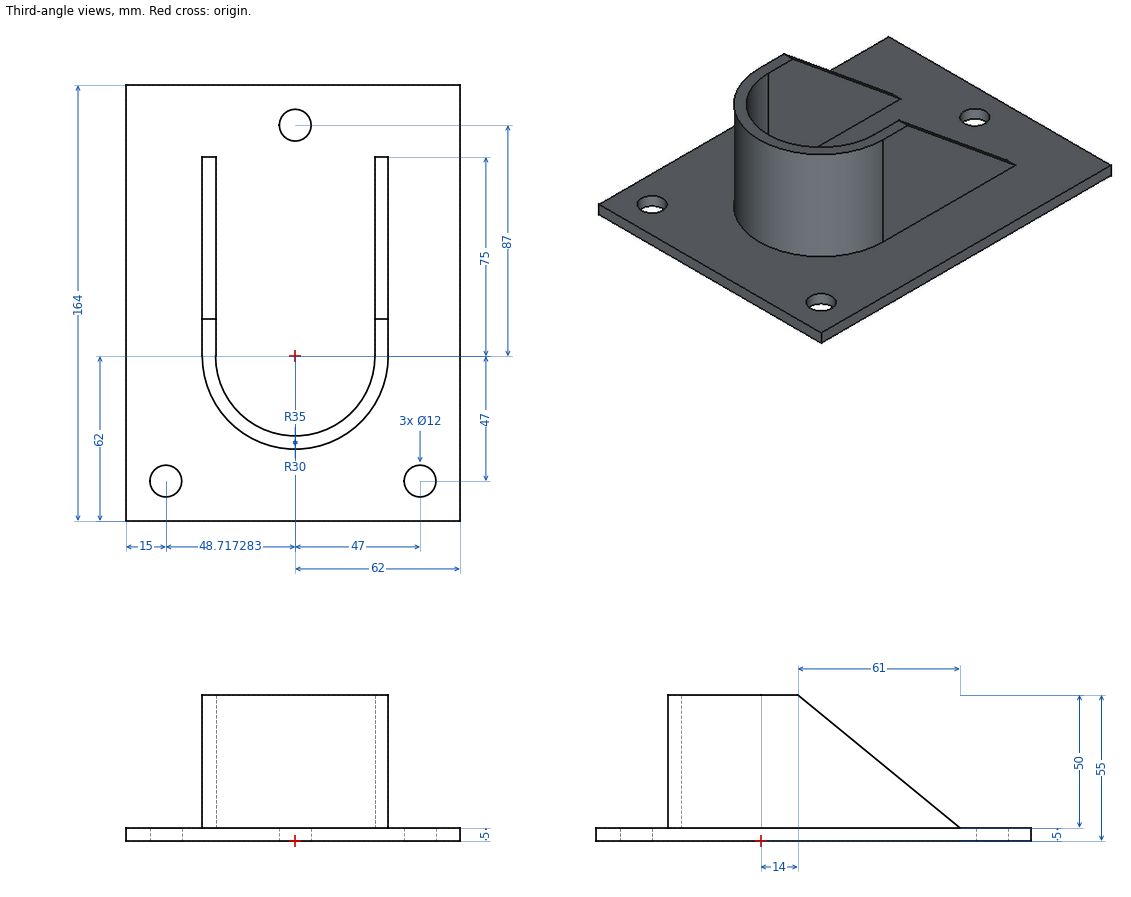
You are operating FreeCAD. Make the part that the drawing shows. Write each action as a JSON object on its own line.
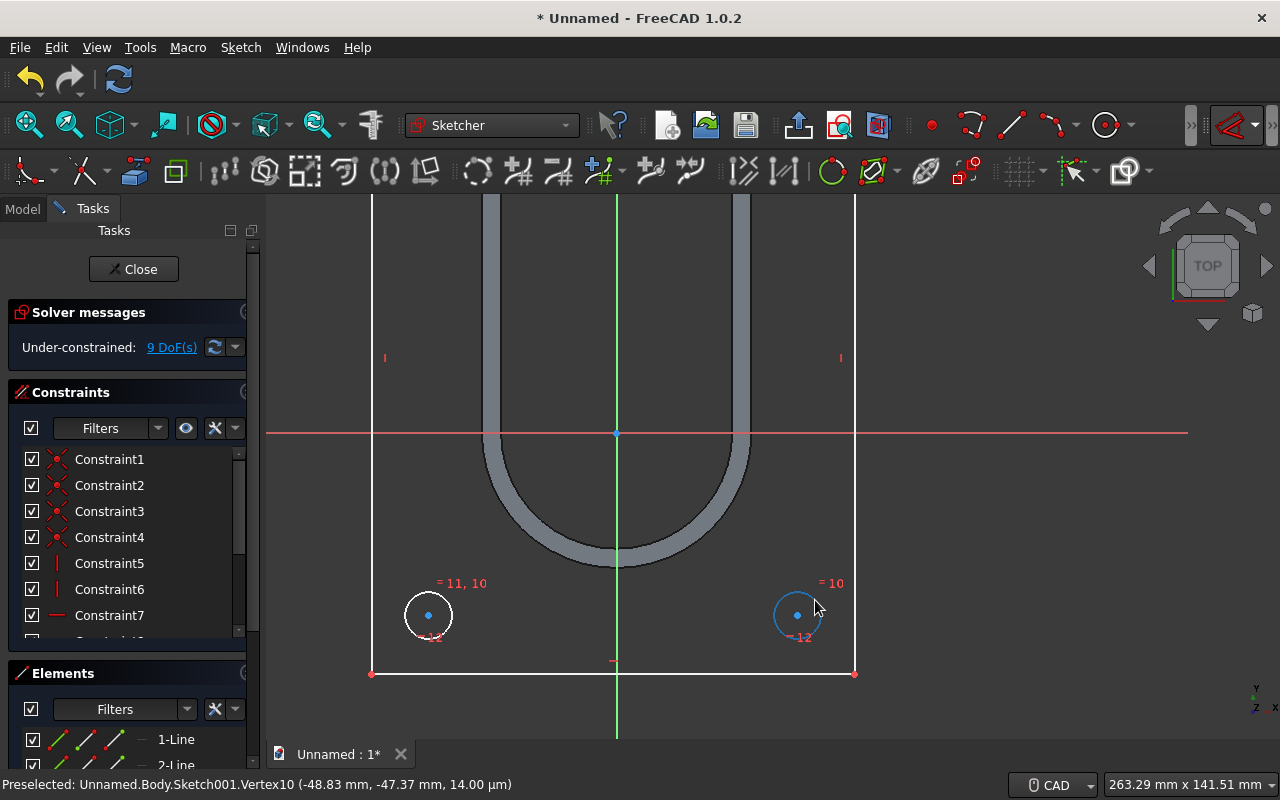
{"action": "left_click", "coordinate": [814, 599]}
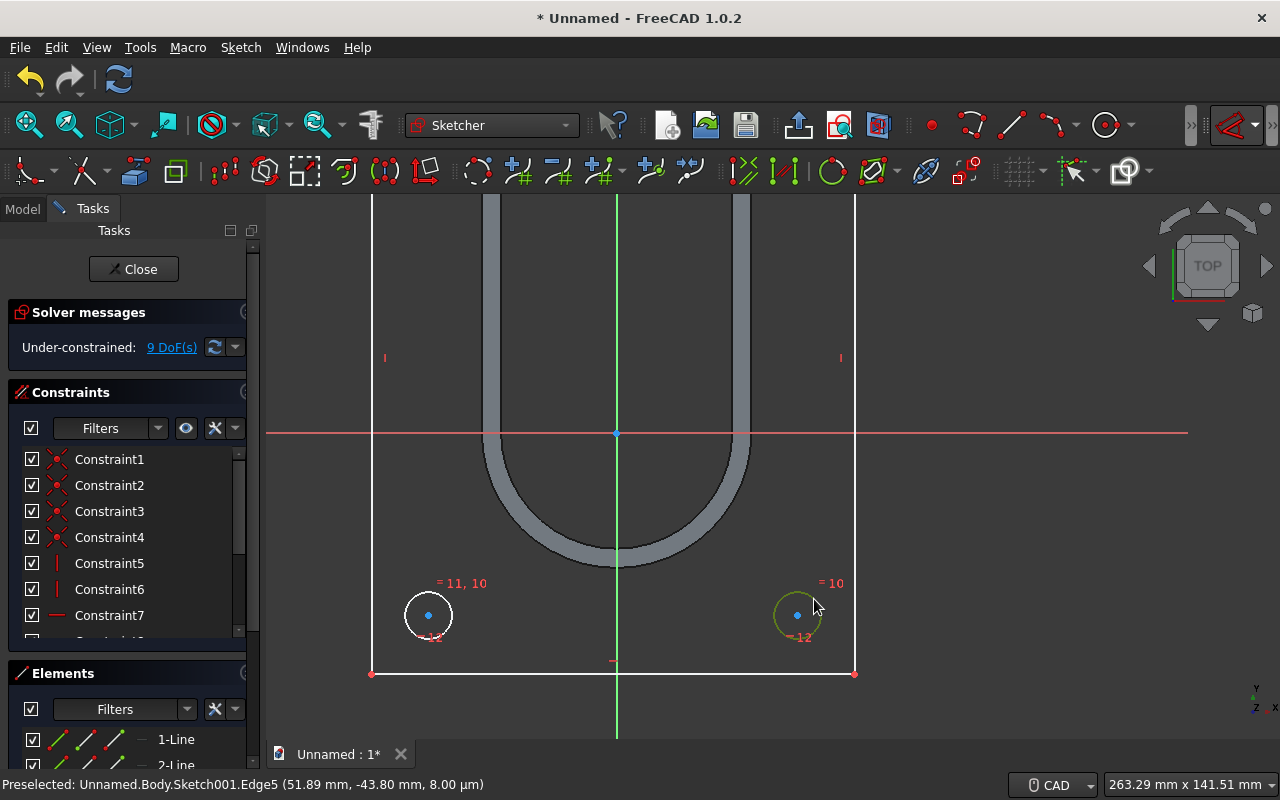
{"action": "left_click", "coordinate": [1258, 126]}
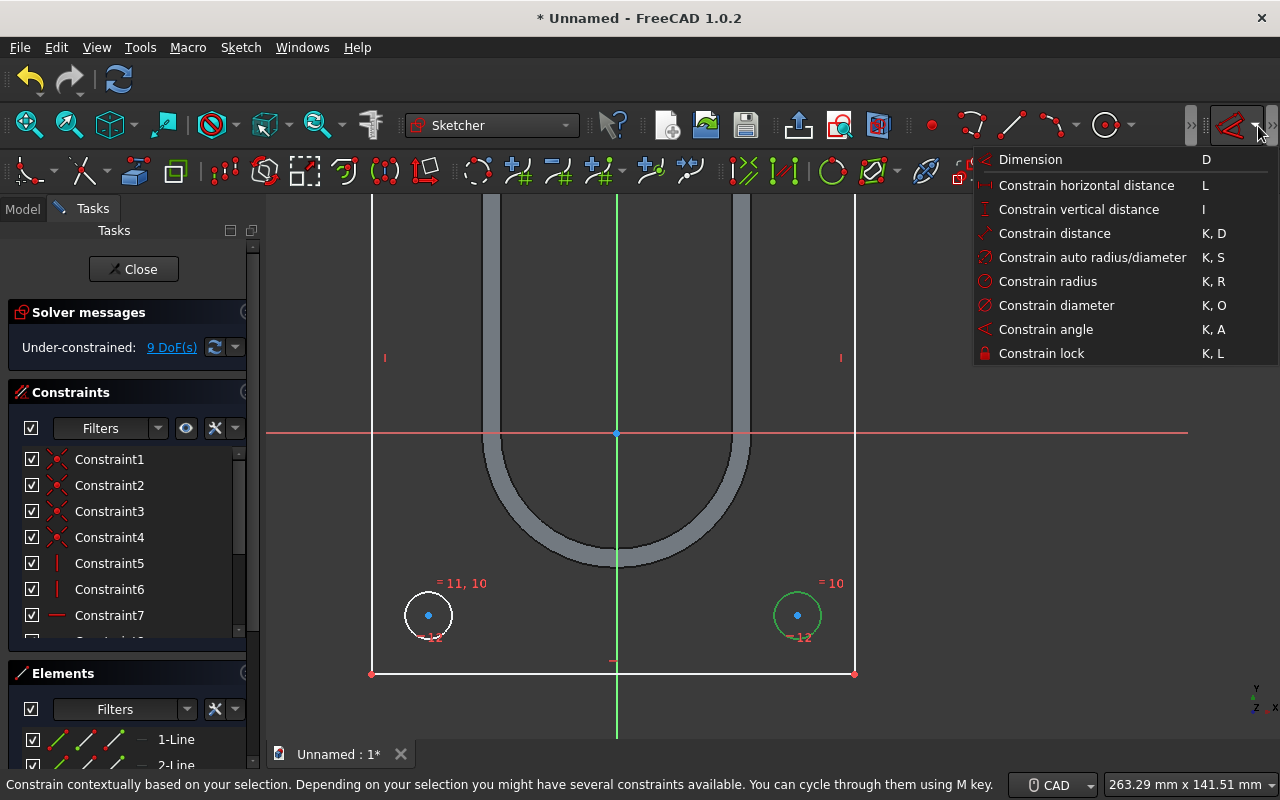
{"action": "left_click", "coordinate": [1126, 305]}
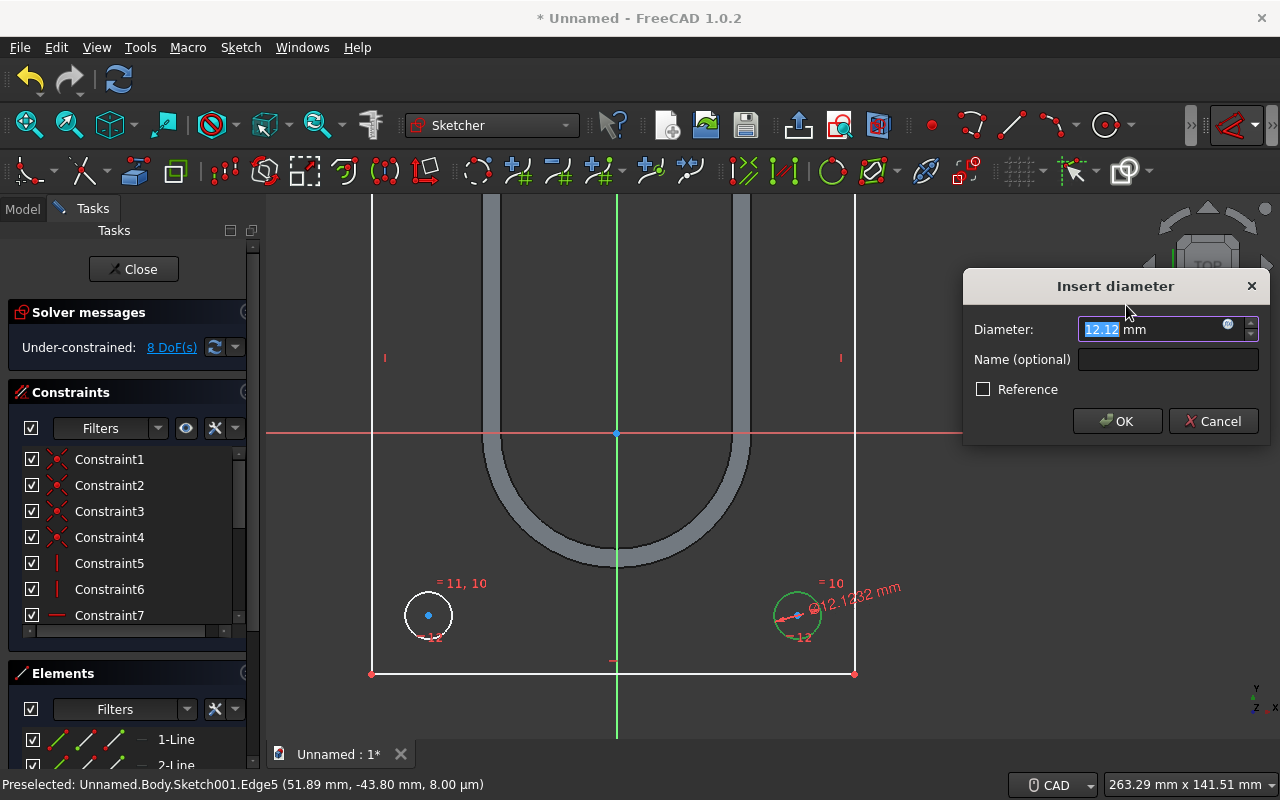
{"action": "type", "text": "12"}
{"action": "key", "text": "Return"}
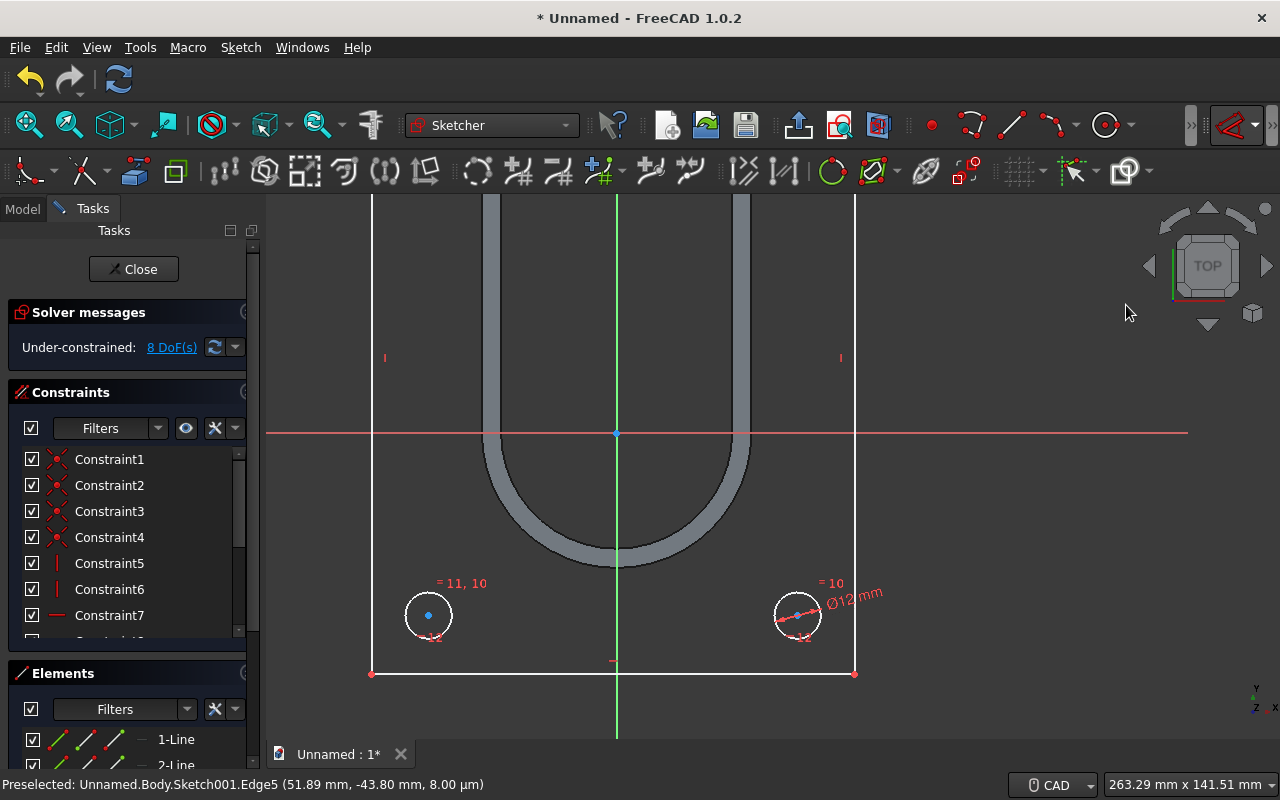
{"action": "left_click", "coordinate": [798, 616]}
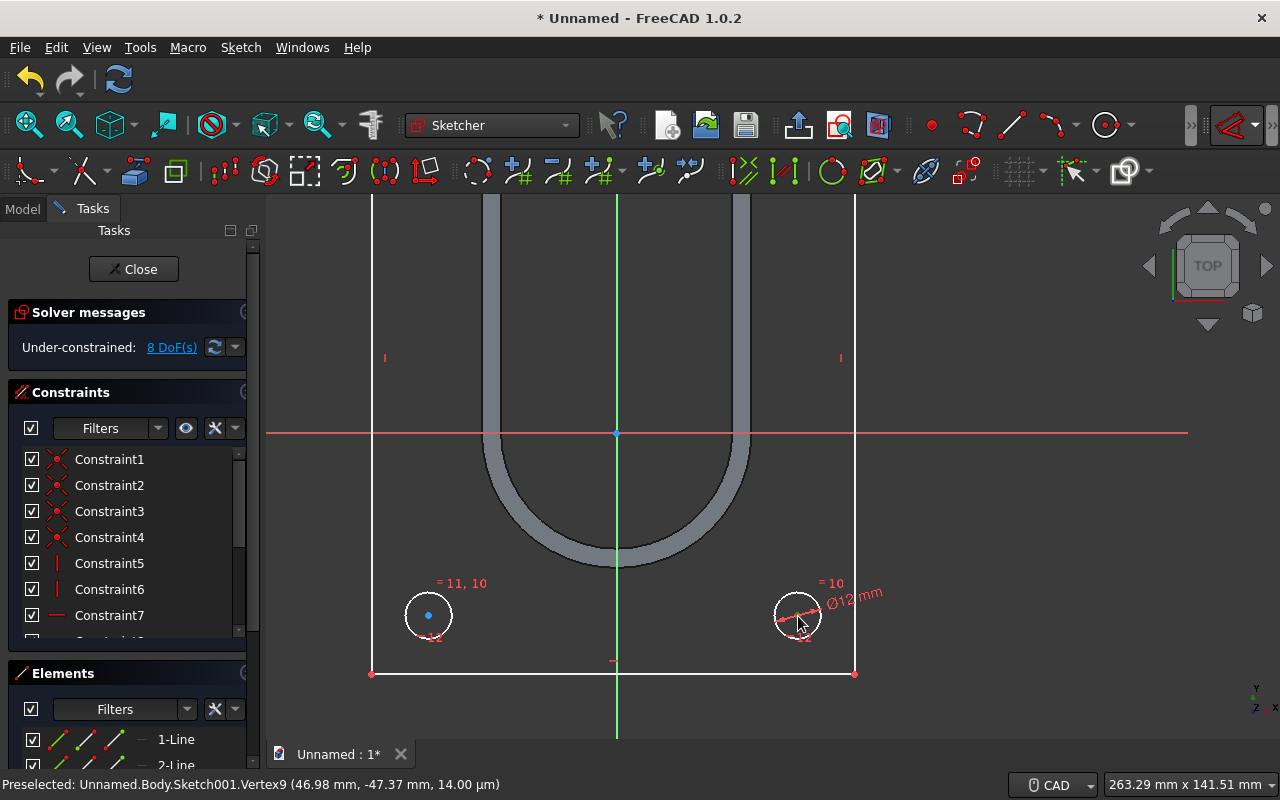
{"action": "key", "text": "l"}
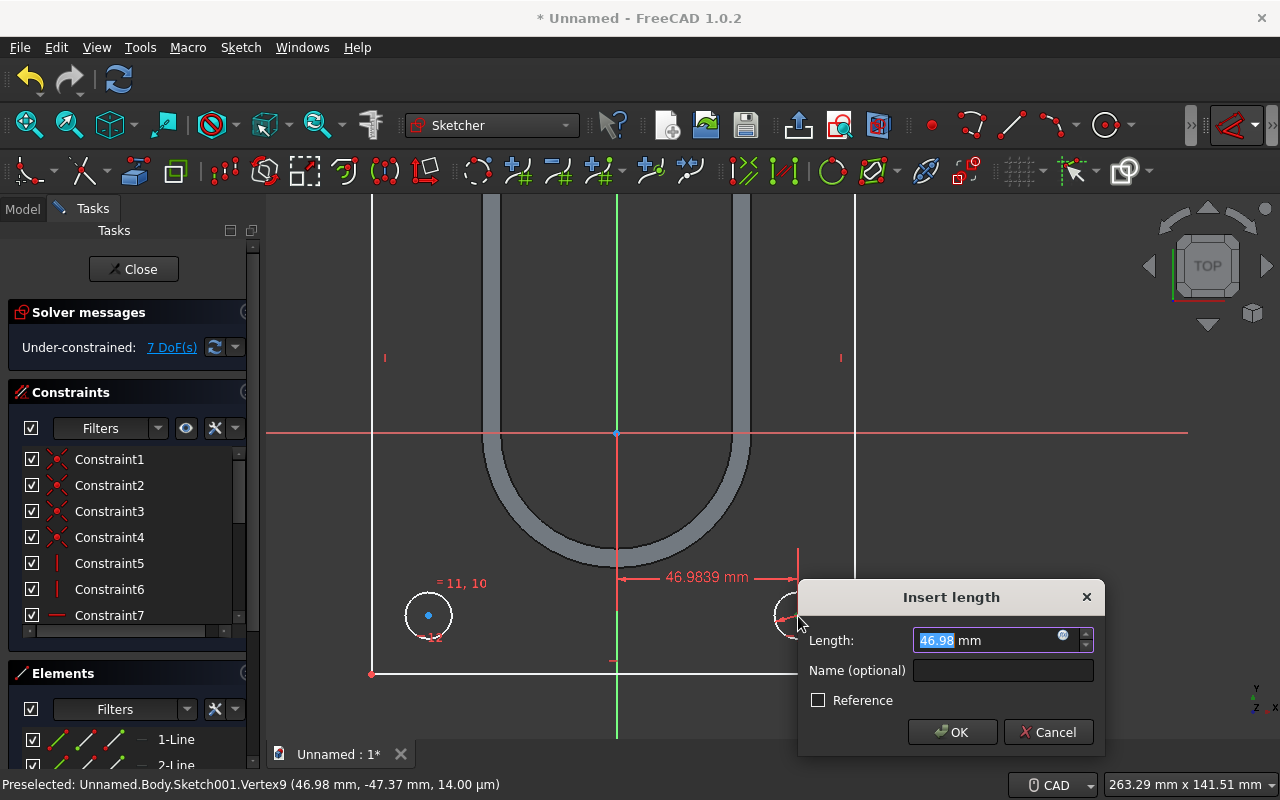
{"action": "type", "text": "47"}
{"action": "key", "text": "Return"}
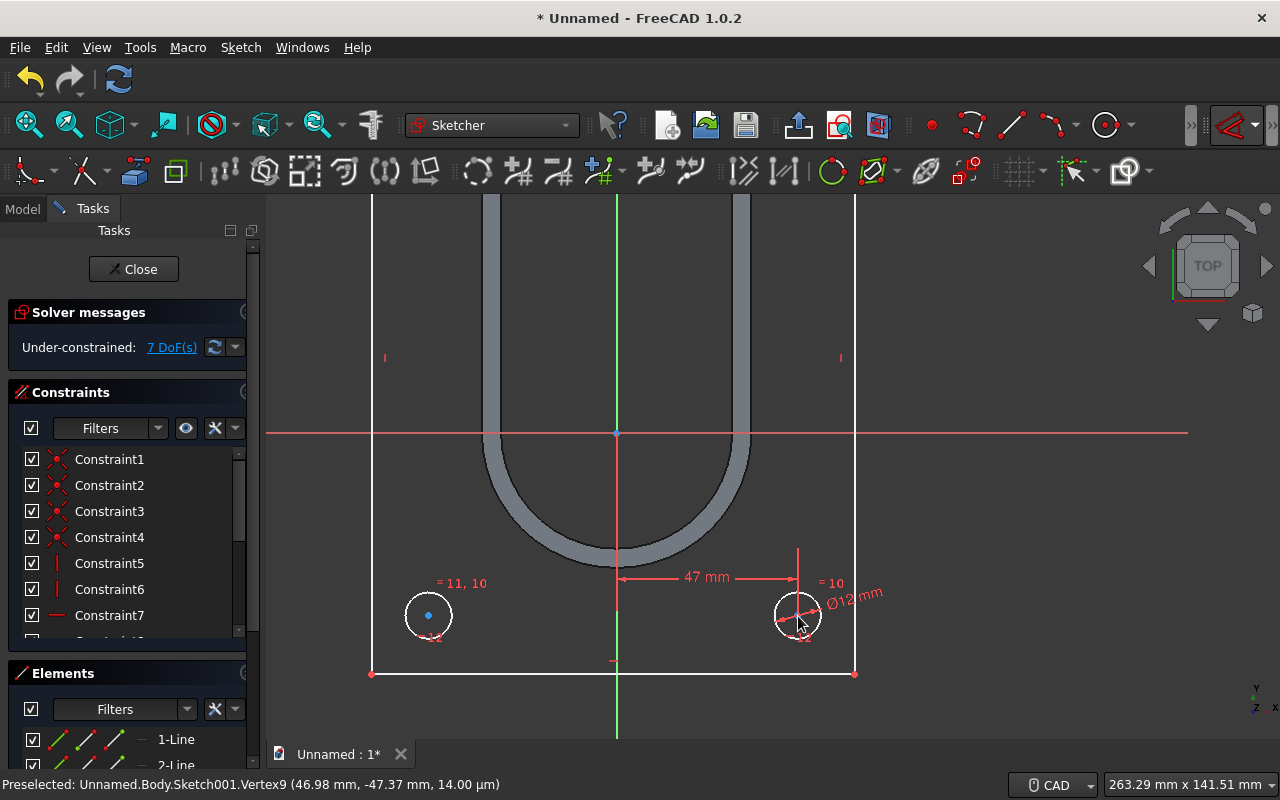
{"action": "left_click", "coordinate": [798, 616]}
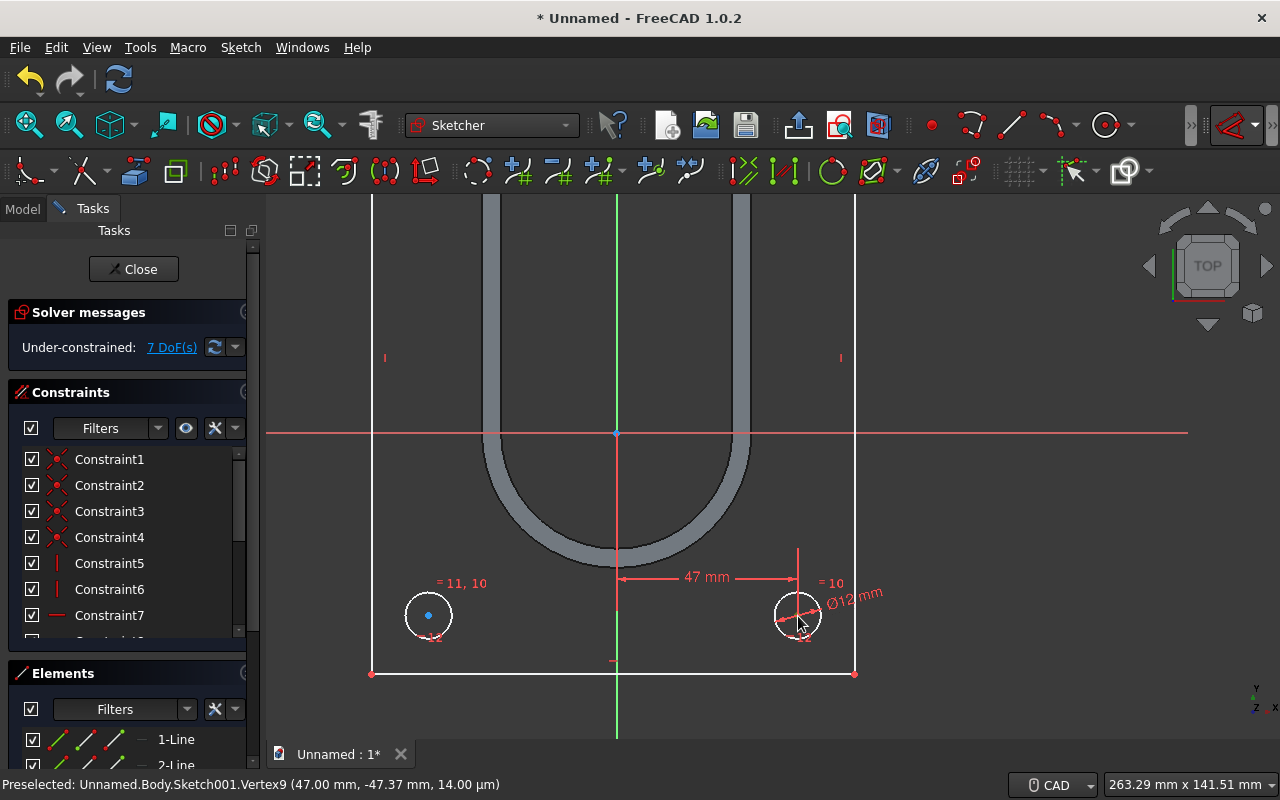
{"action": "key", "text": "i"}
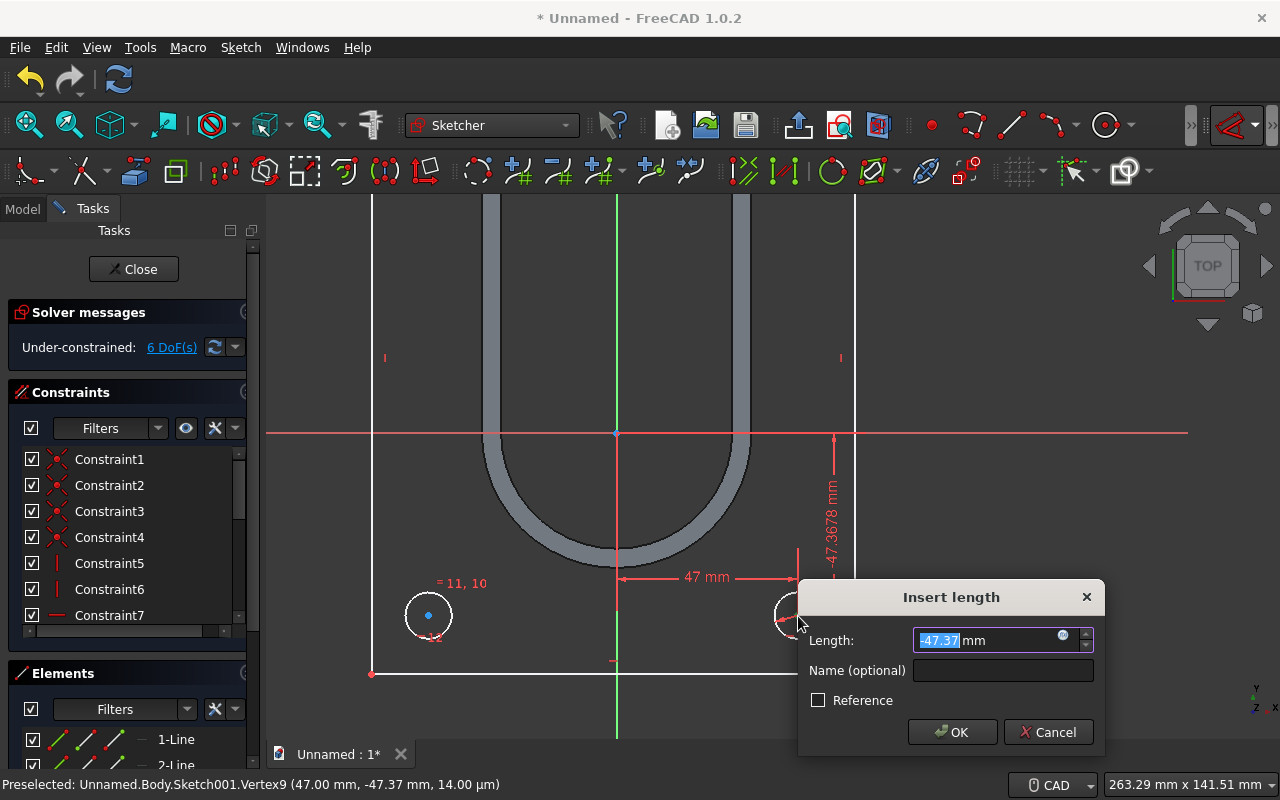
{"action": "type", "text": "-47"}
{"action": "key", "text": "Return"}